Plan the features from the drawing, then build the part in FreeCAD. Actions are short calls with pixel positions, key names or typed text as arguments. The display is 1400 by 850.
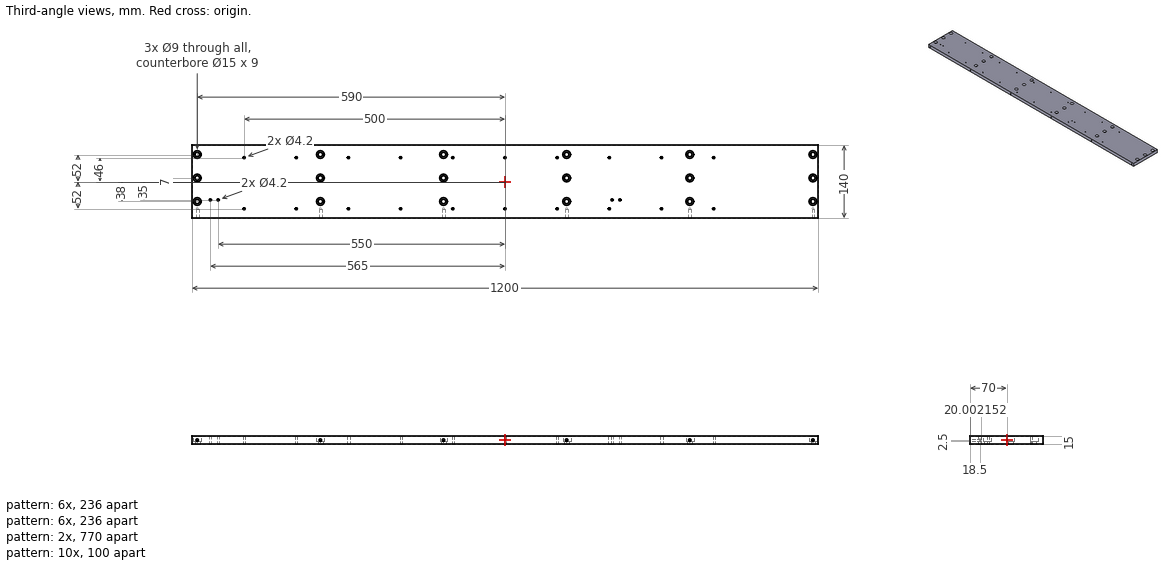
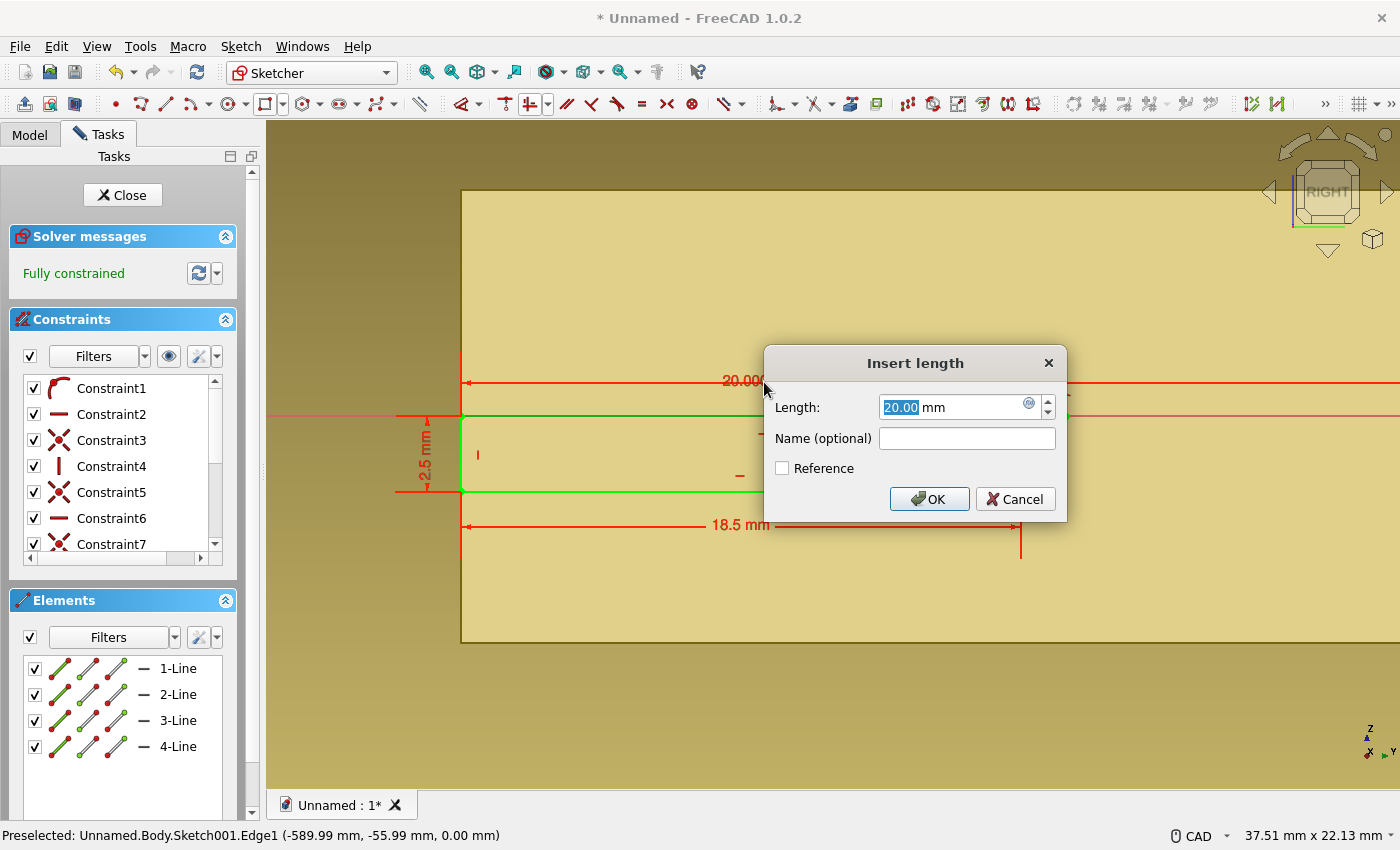
text(20.002152)
key(Return)
key(Escape)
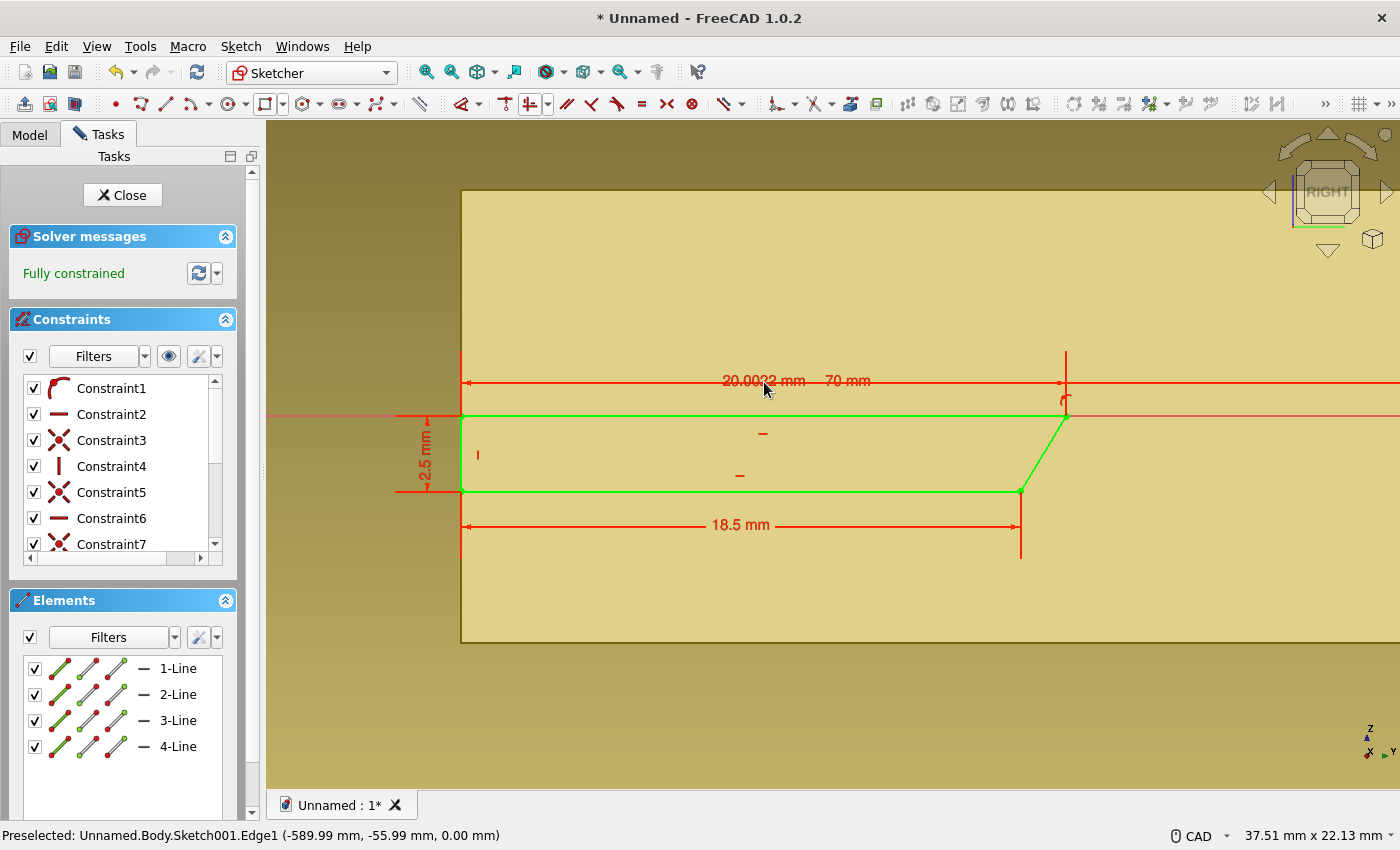
click(123, 195)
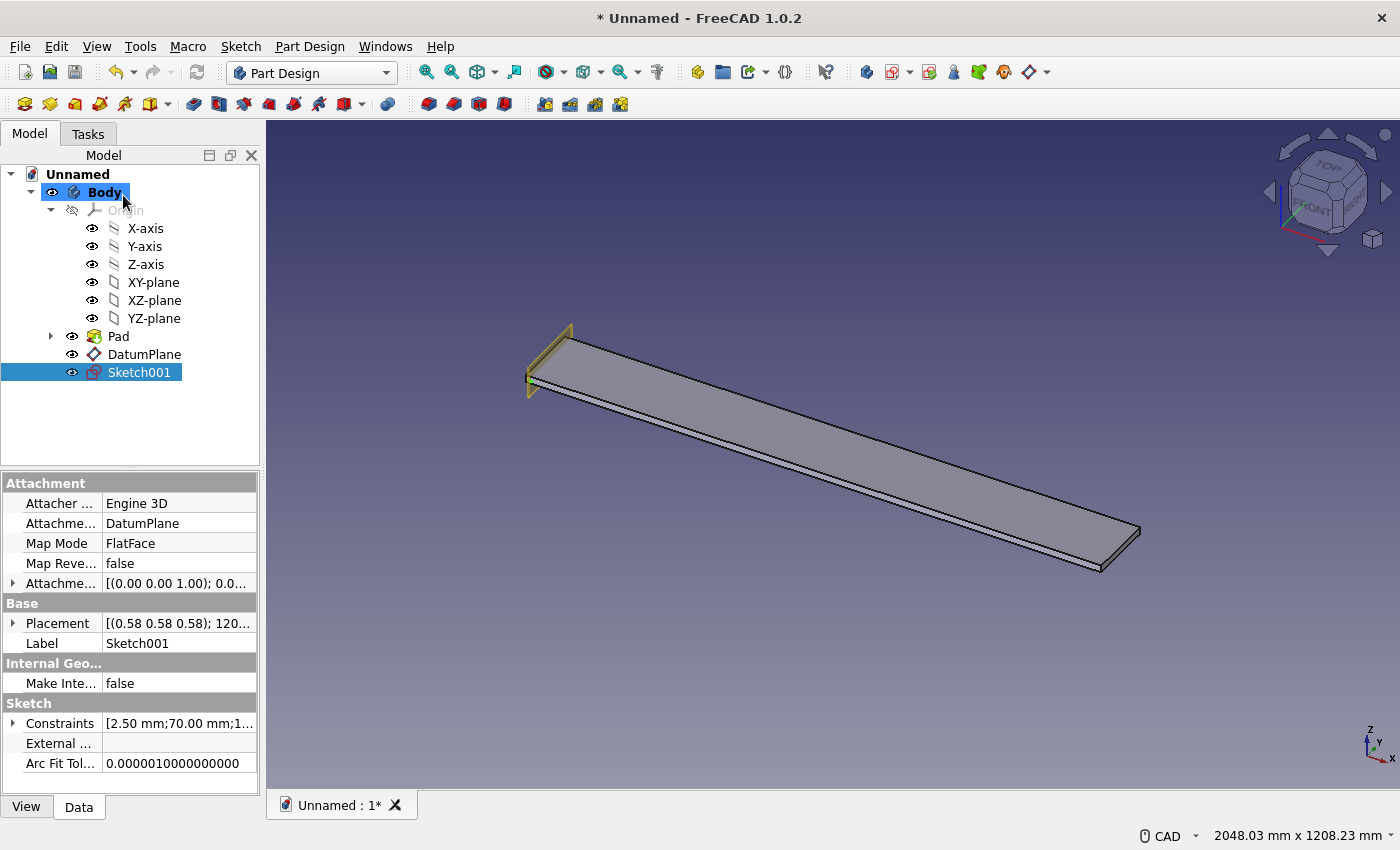
click(244, 104)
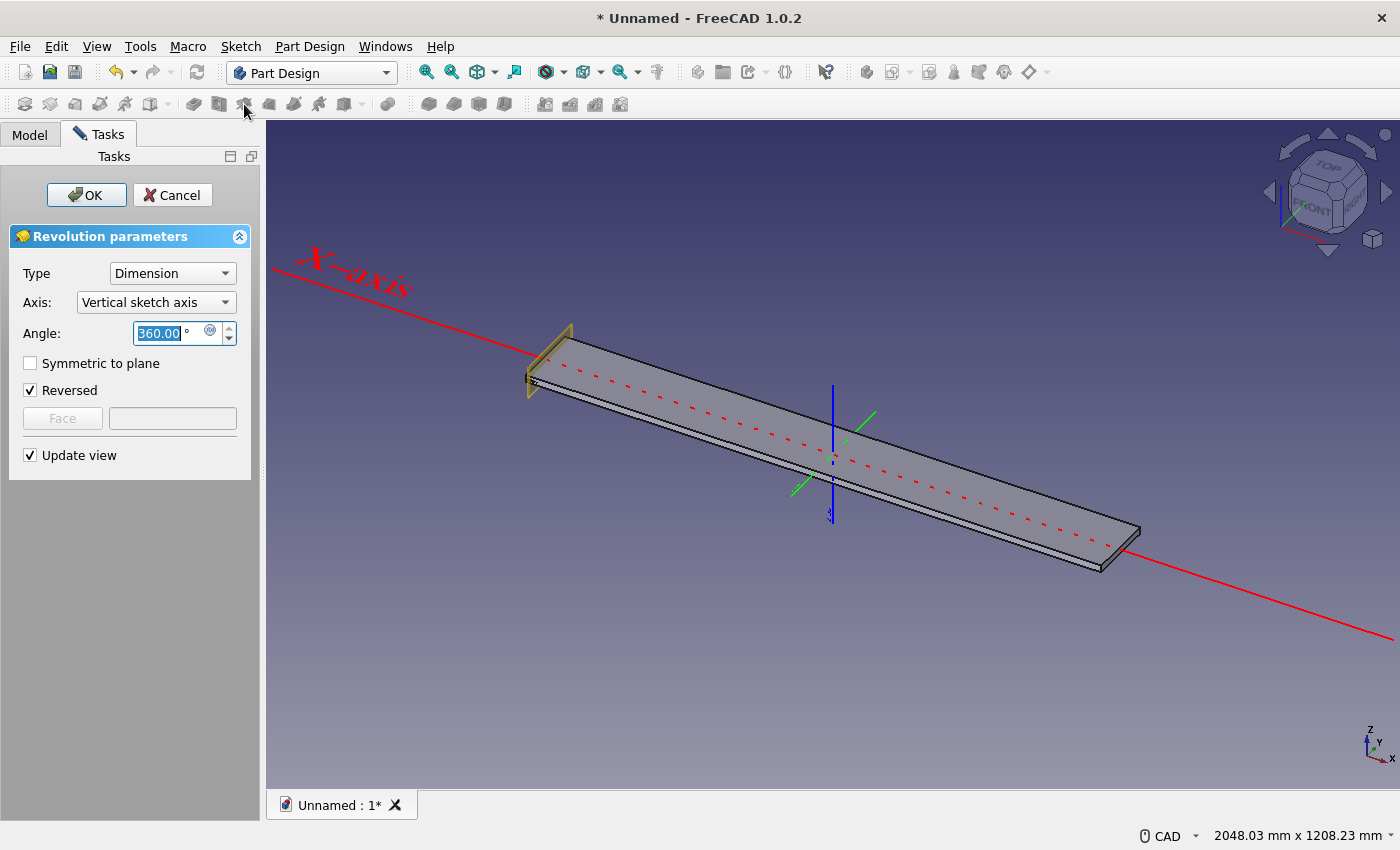
click(157, 302)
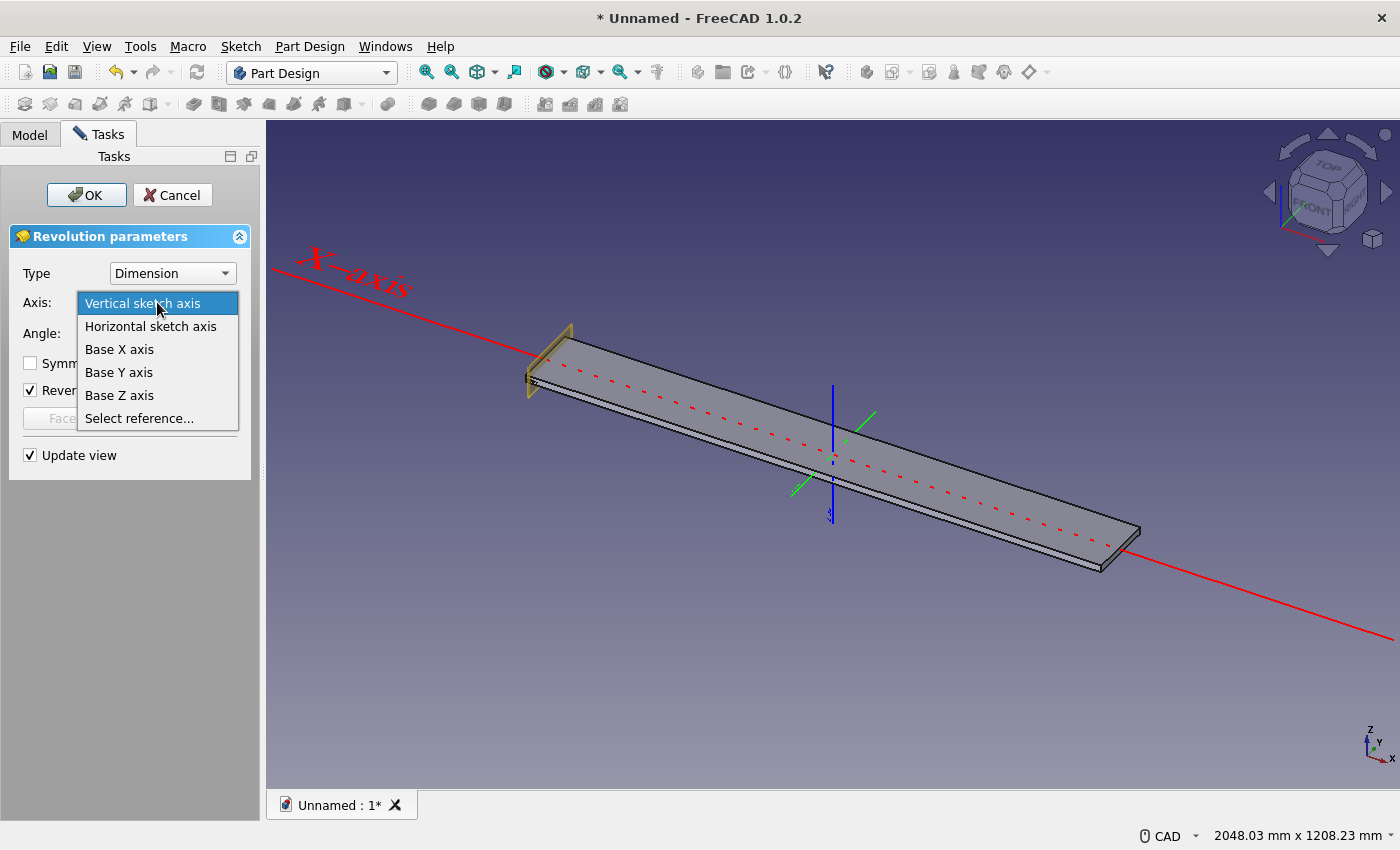
click(156, 326)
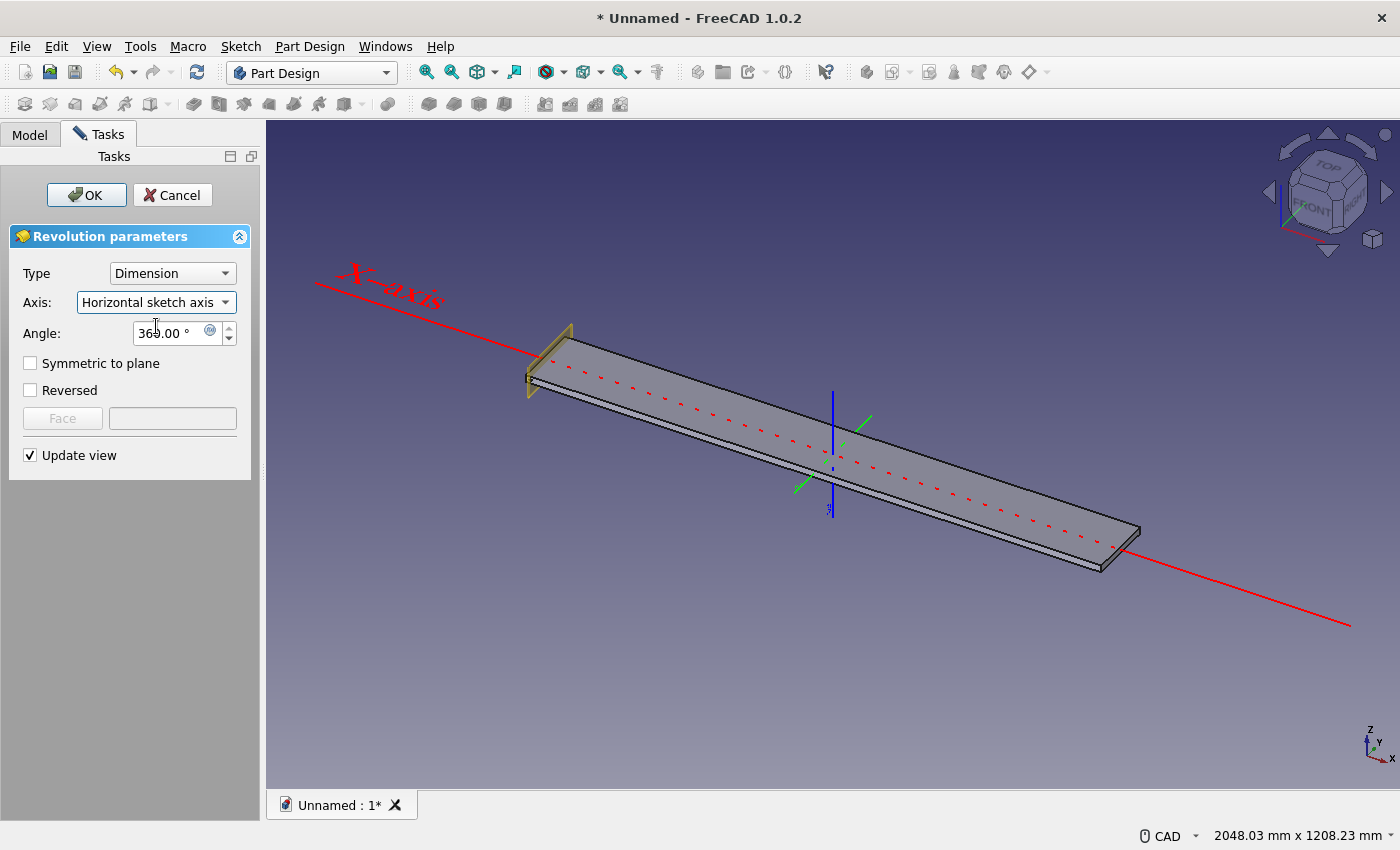
click(87, 195)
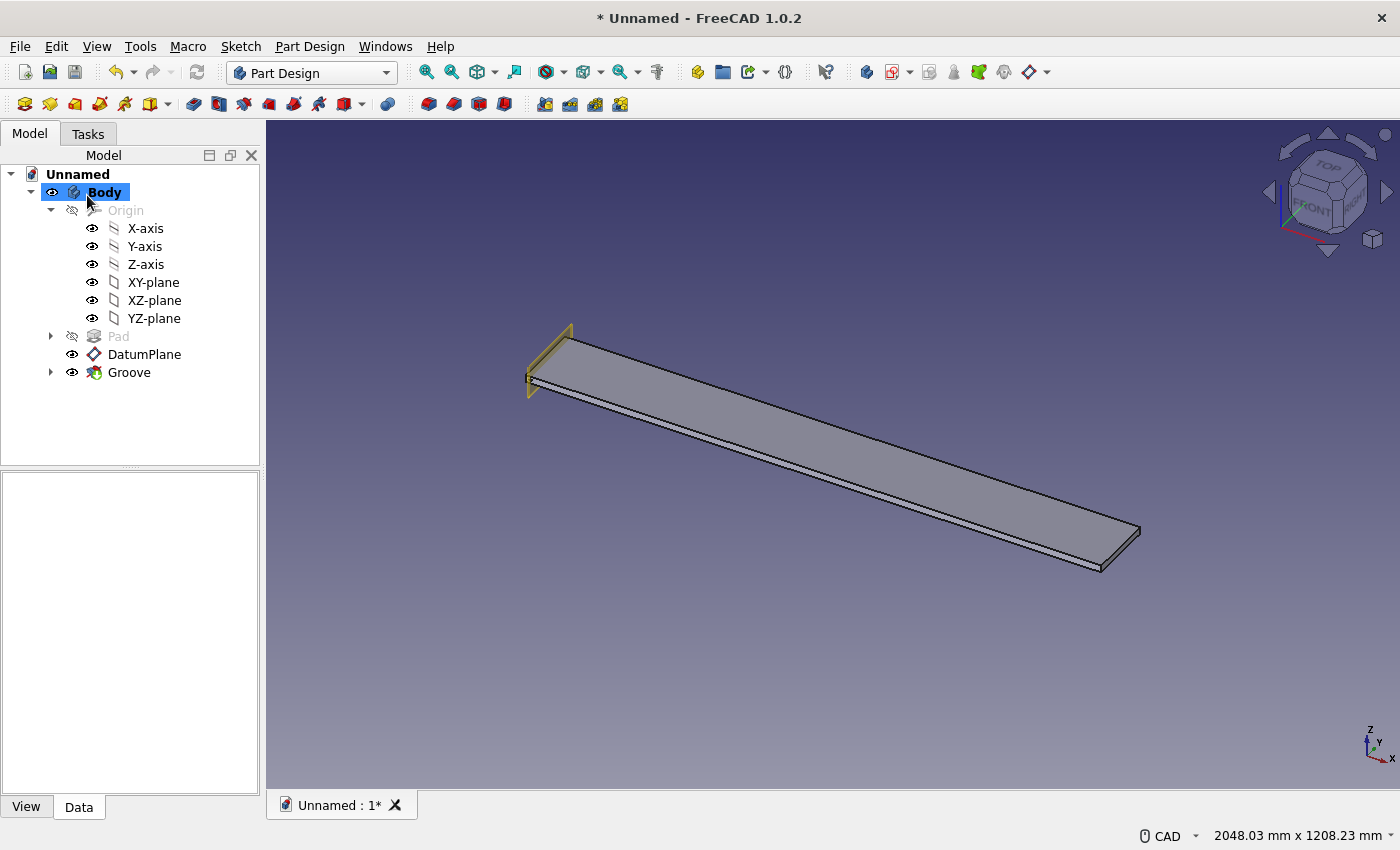
click(117, 354)
key(space)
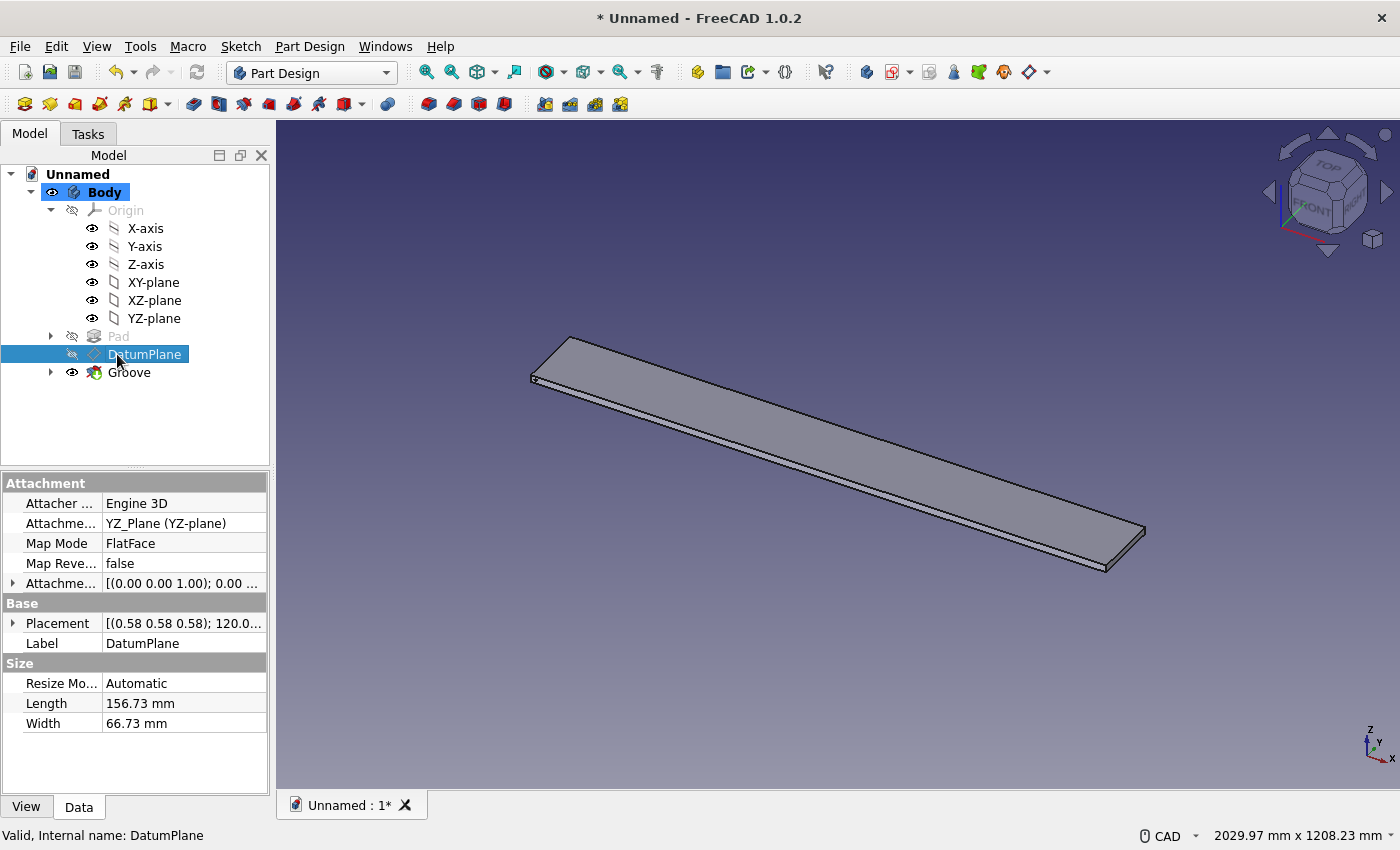
click(117, 372)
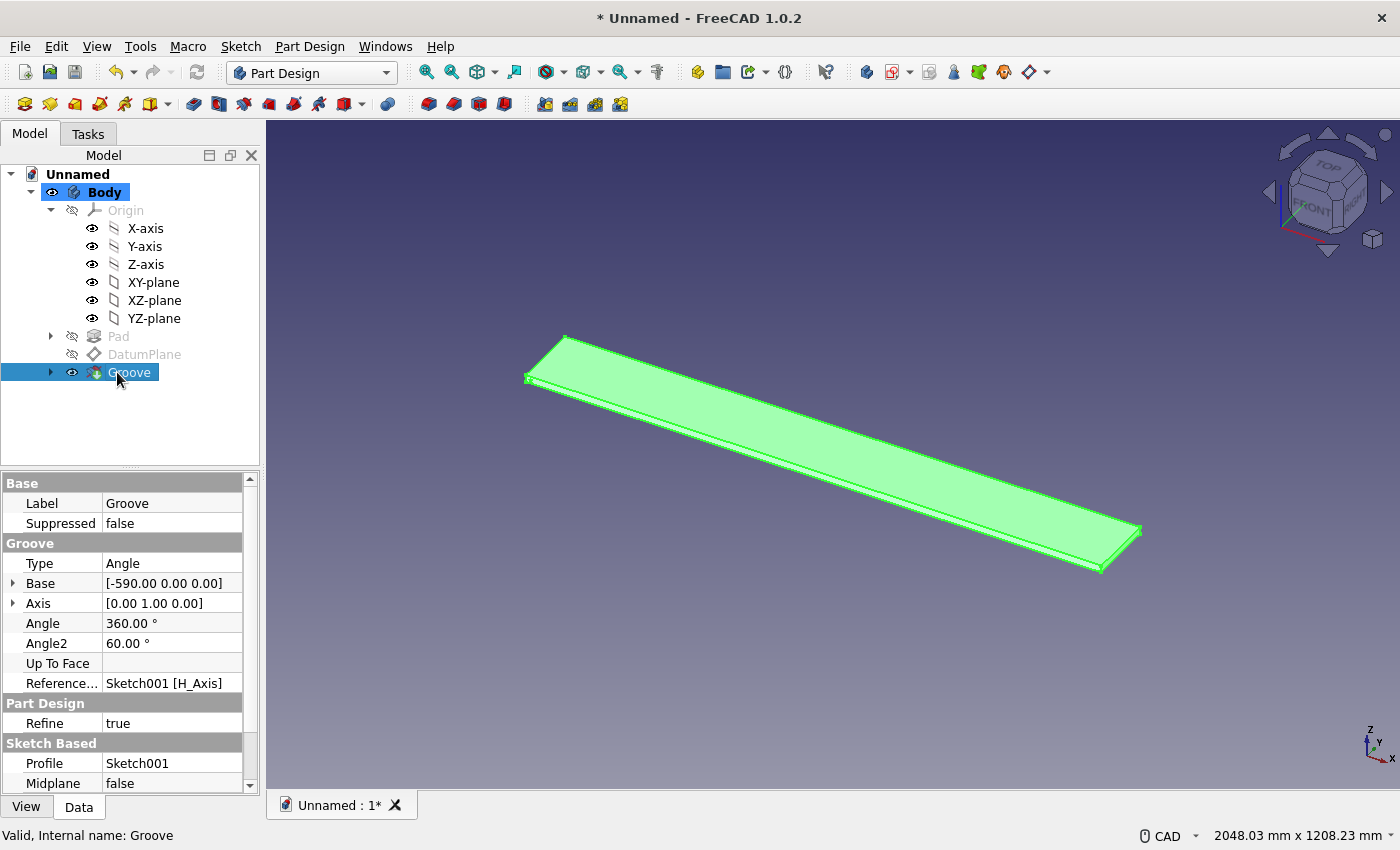
click(570, 104)